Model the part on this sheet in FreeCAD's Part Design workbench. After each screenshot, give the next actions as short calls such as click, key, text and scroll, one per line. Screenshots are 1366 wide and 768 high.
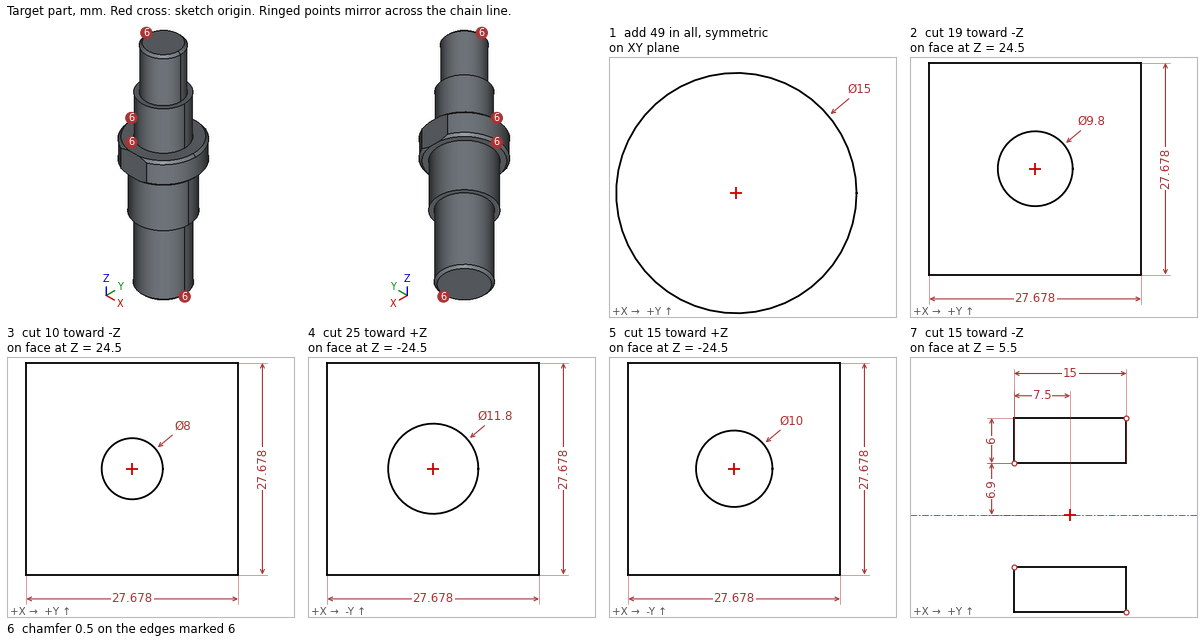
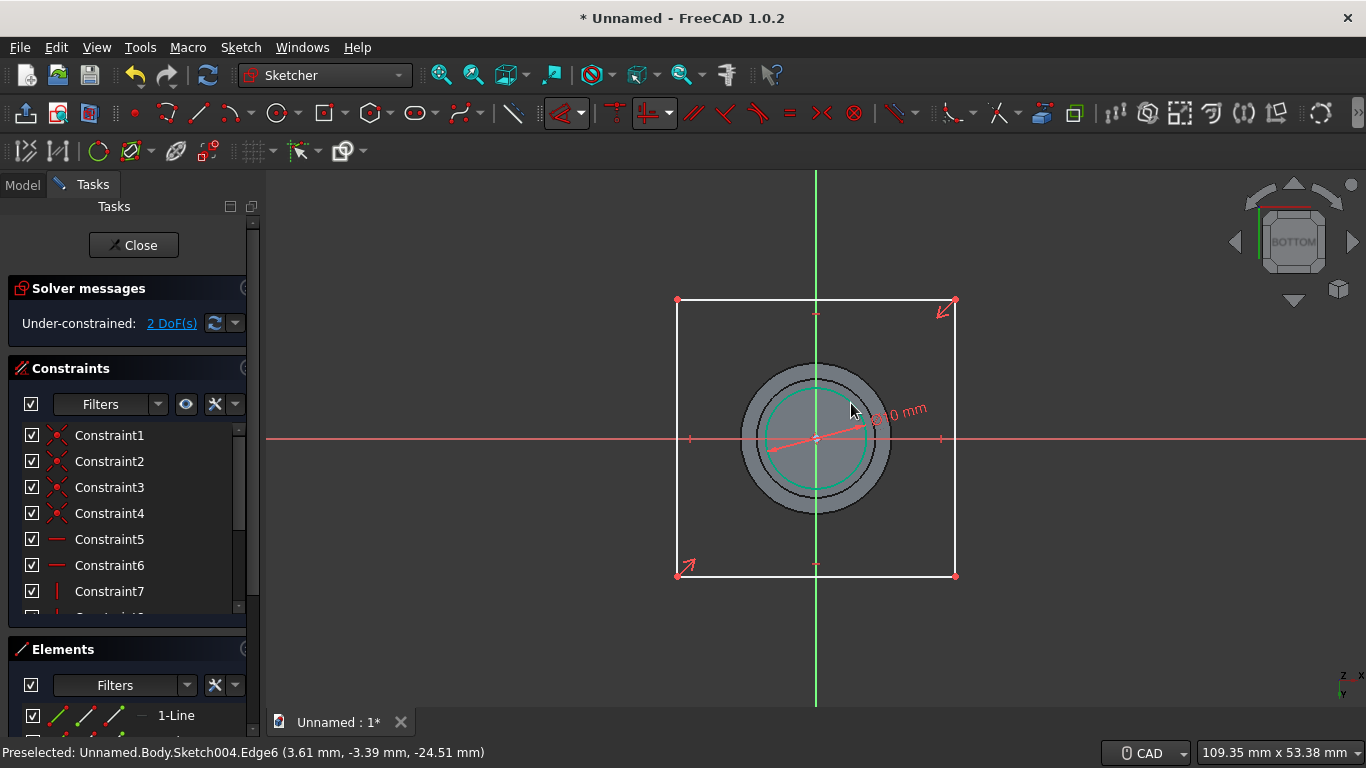
click(760, 577)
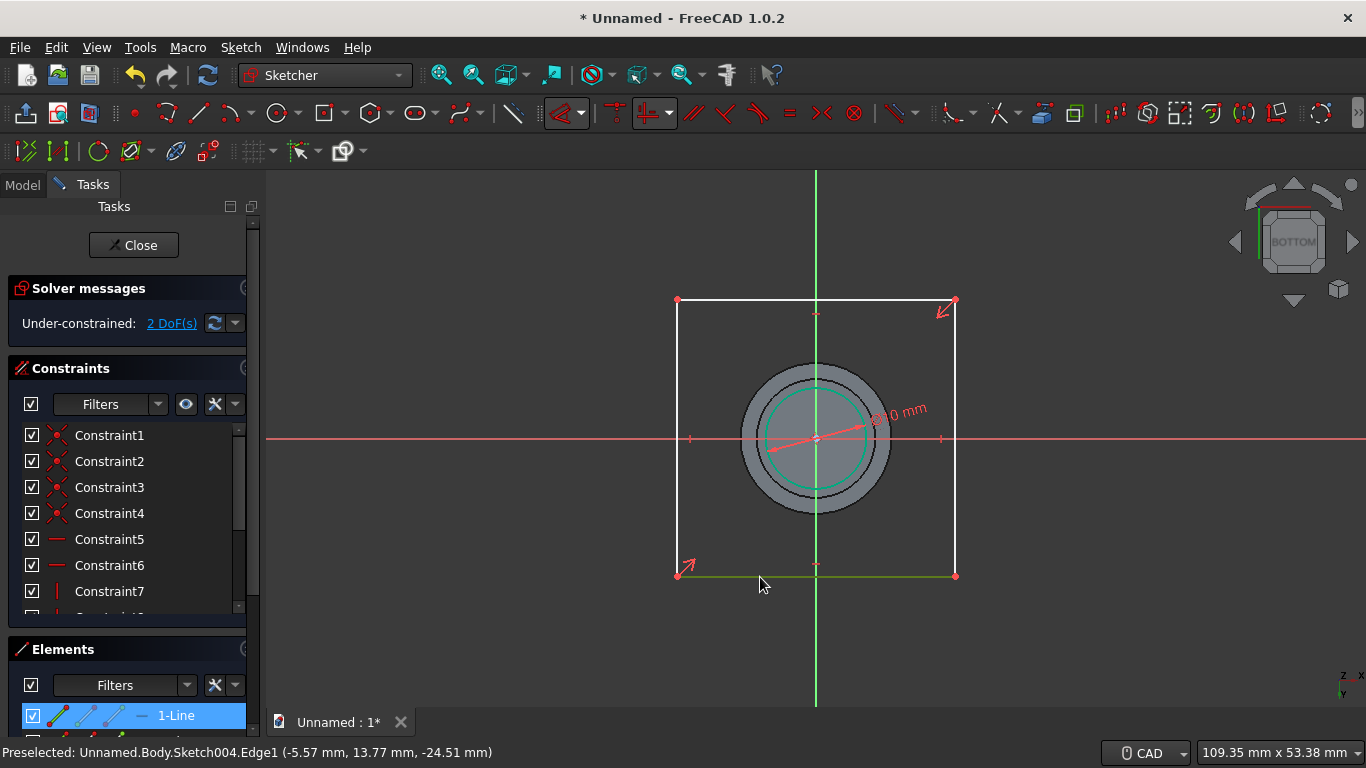
click(584, 114)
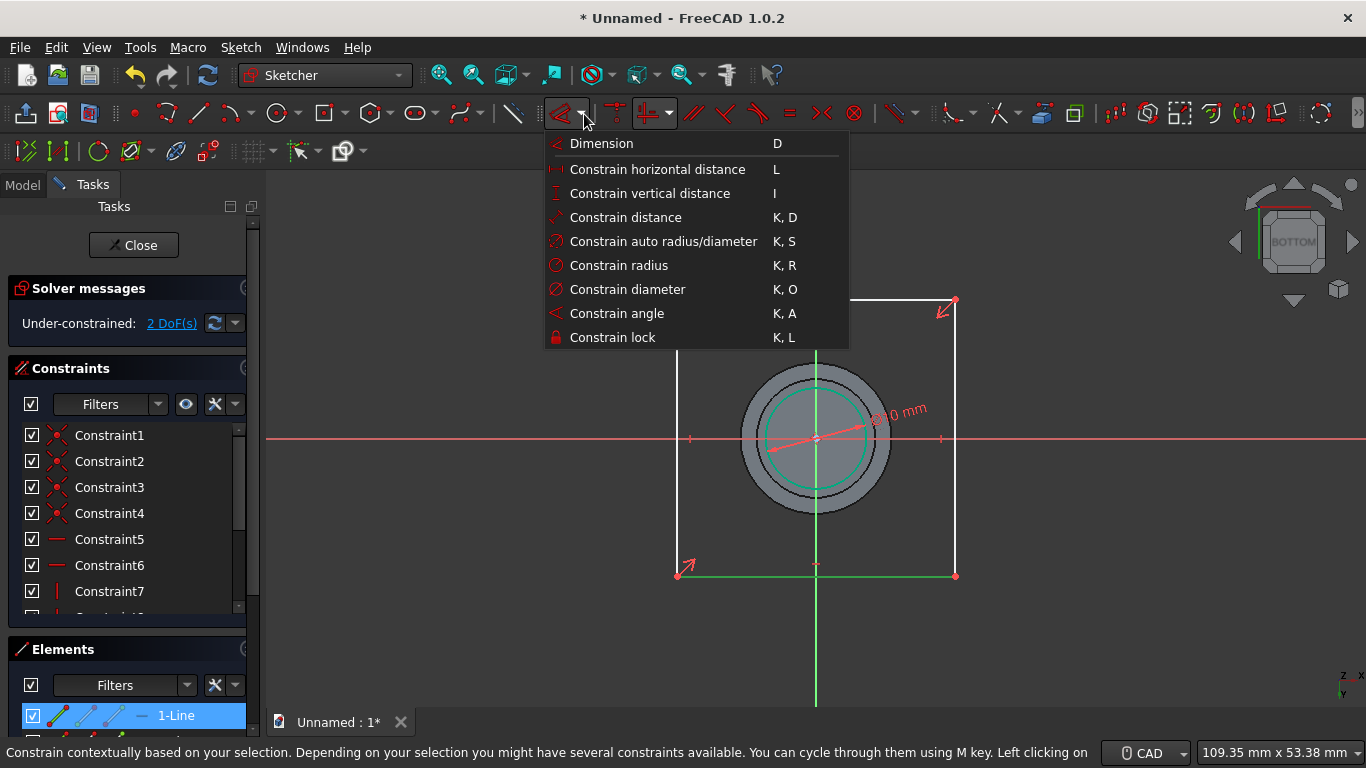
click(697, 169)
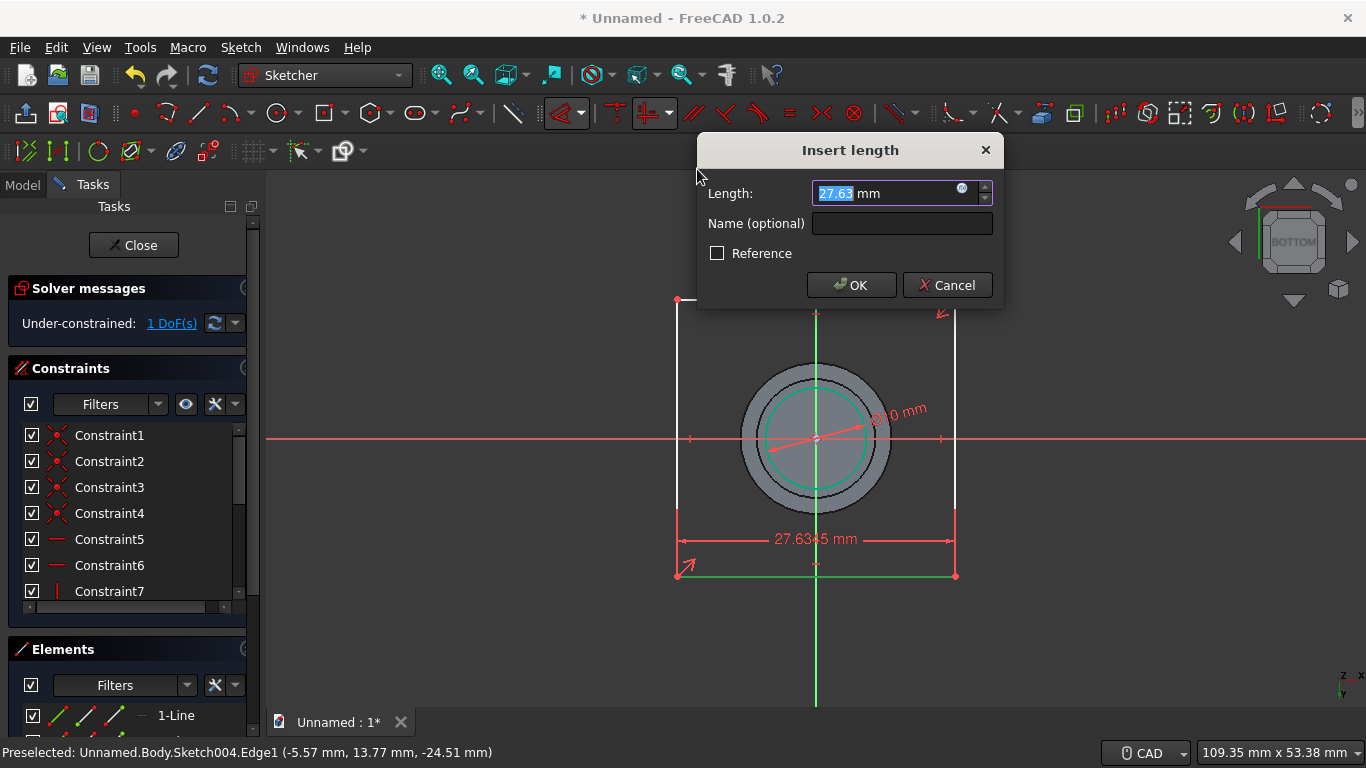
text(27.678)
key(Return)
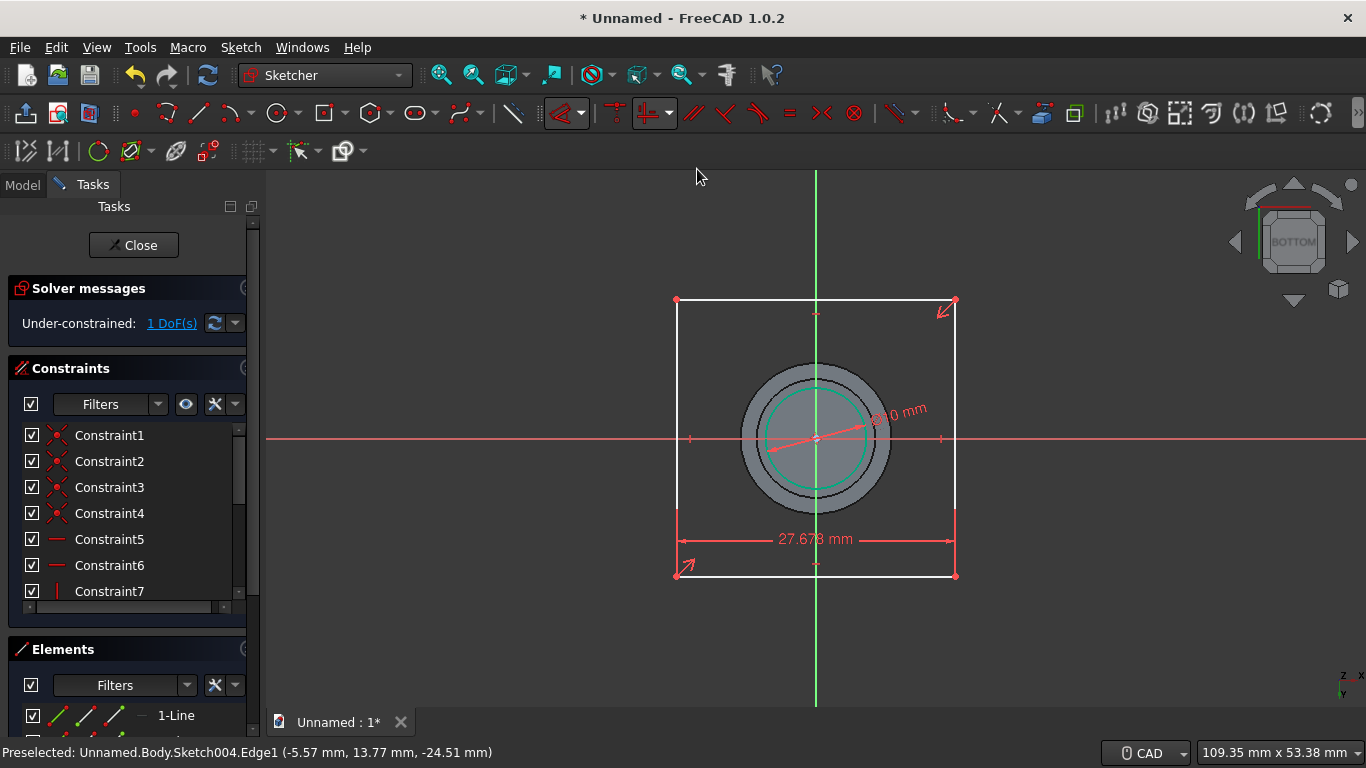
click(955, 494)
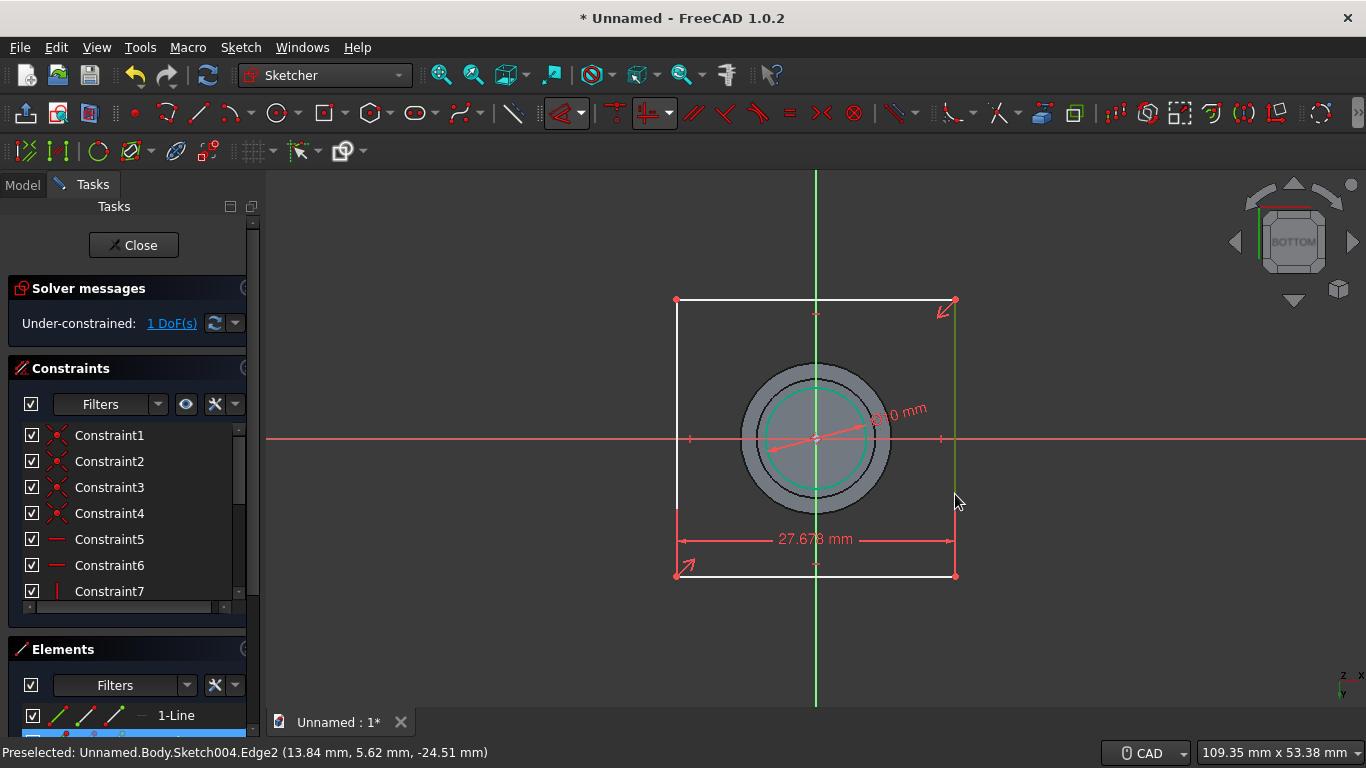
key(i)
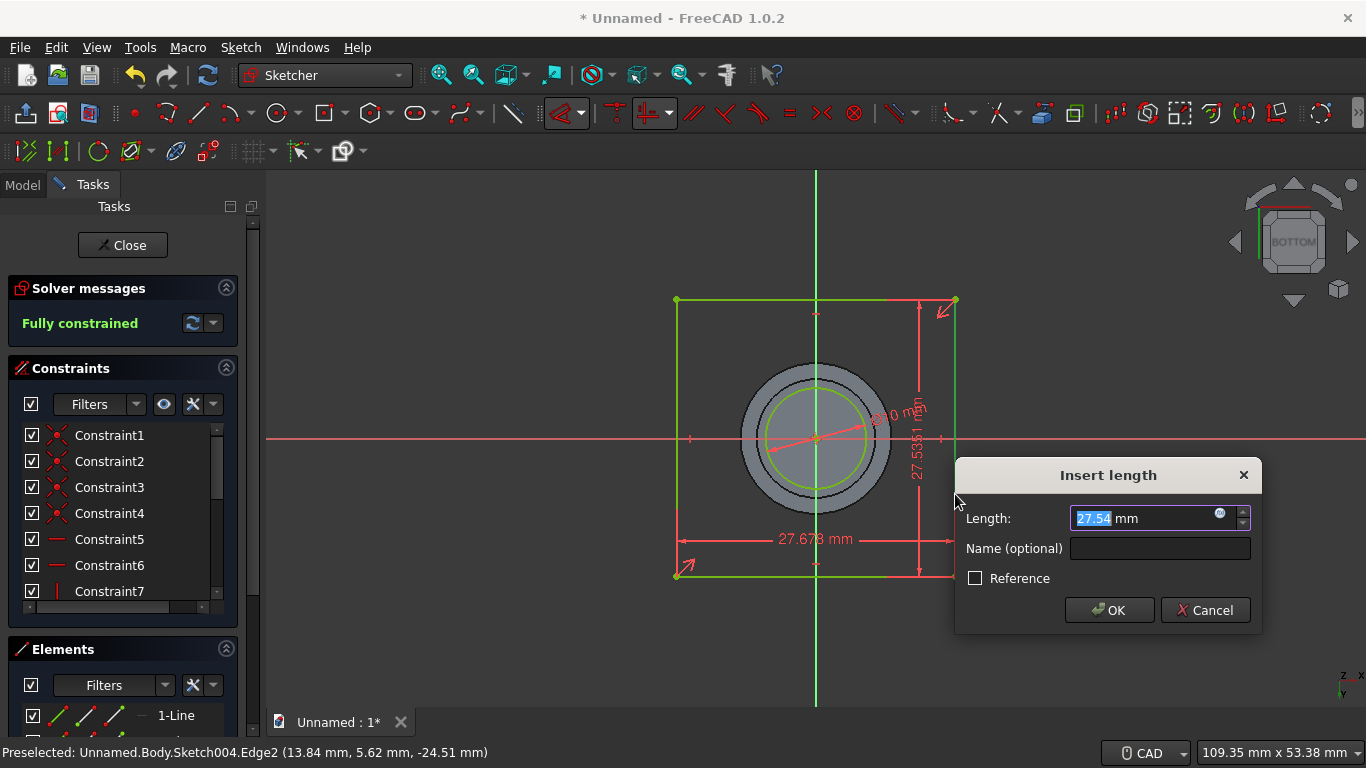
text(27.678)
key(Return)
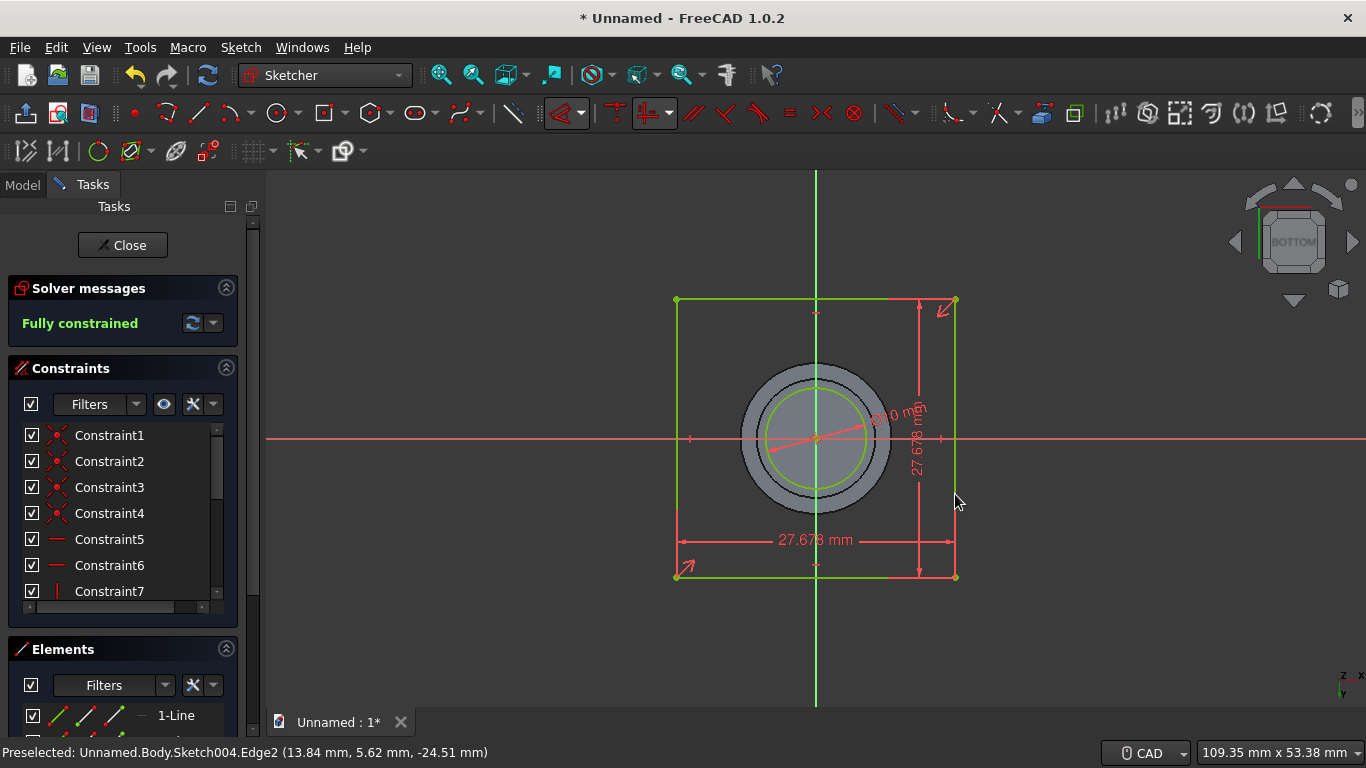
click(123, 245)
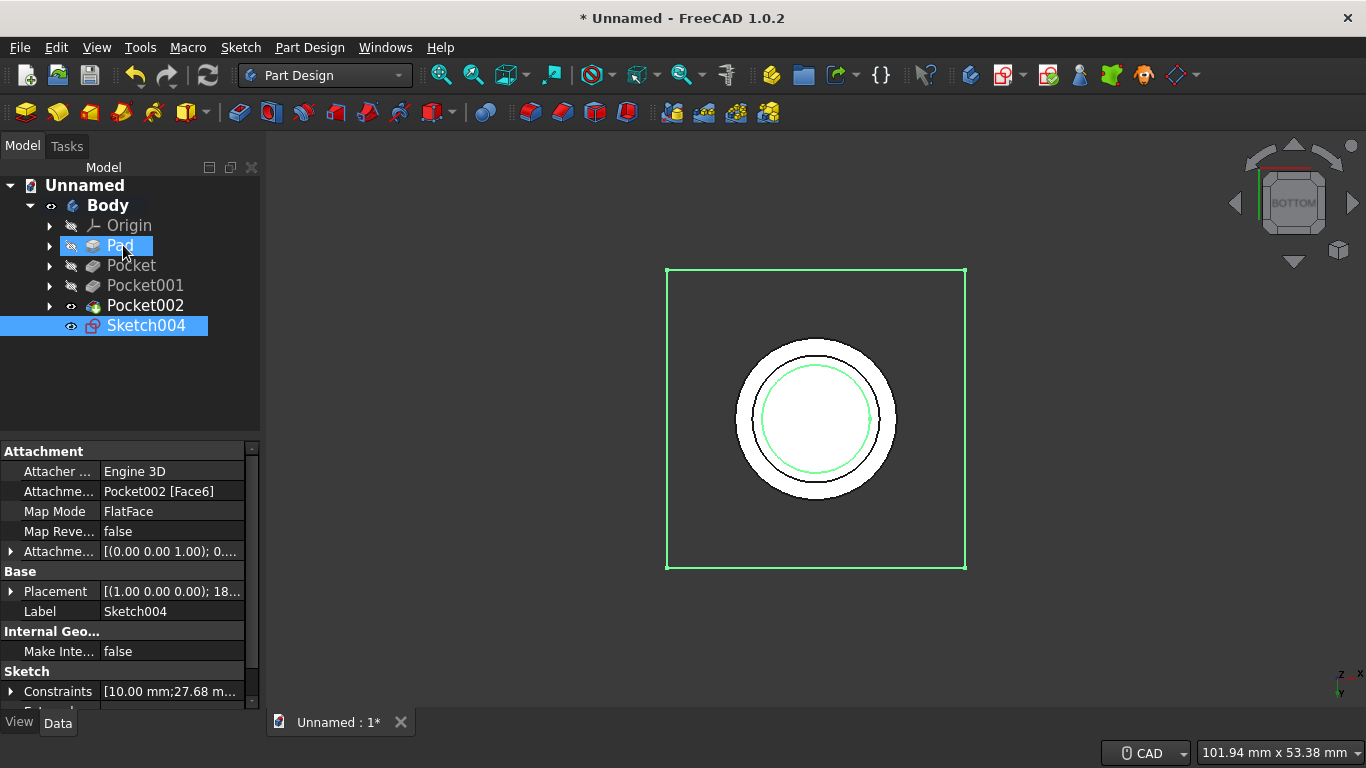
click(240, 112)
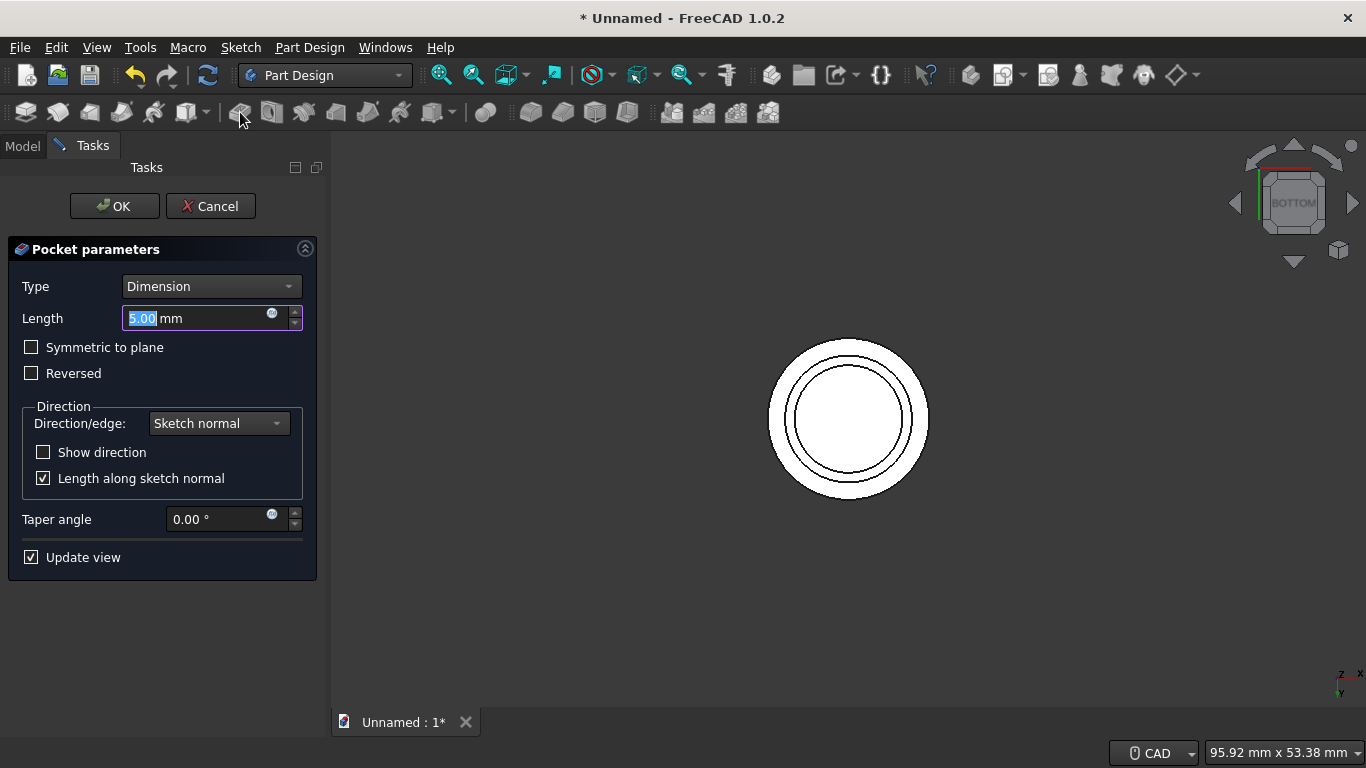
text(15)
key(Tab)